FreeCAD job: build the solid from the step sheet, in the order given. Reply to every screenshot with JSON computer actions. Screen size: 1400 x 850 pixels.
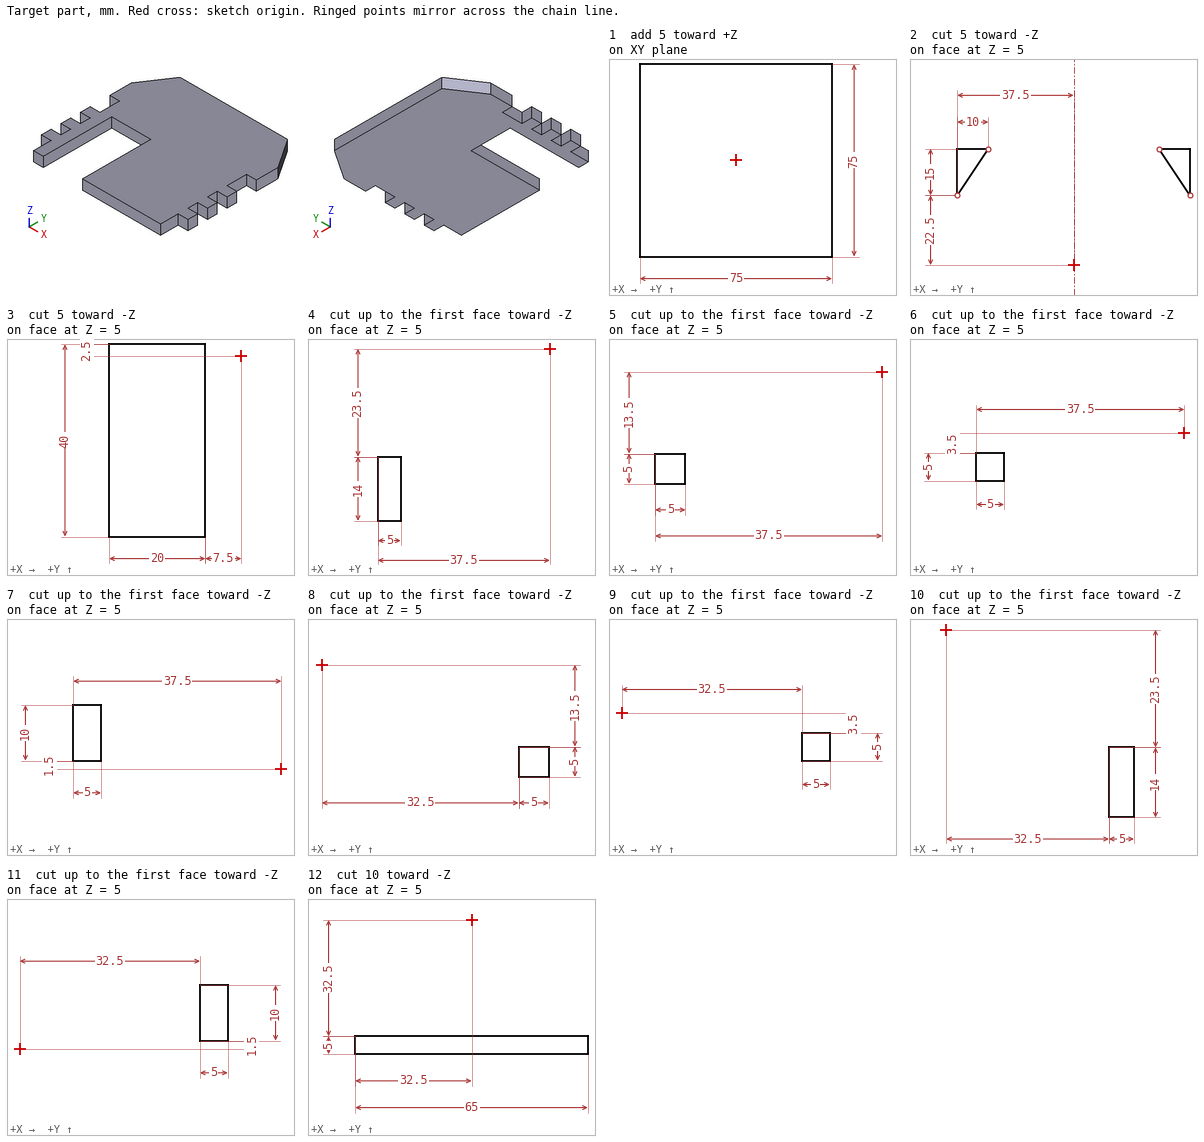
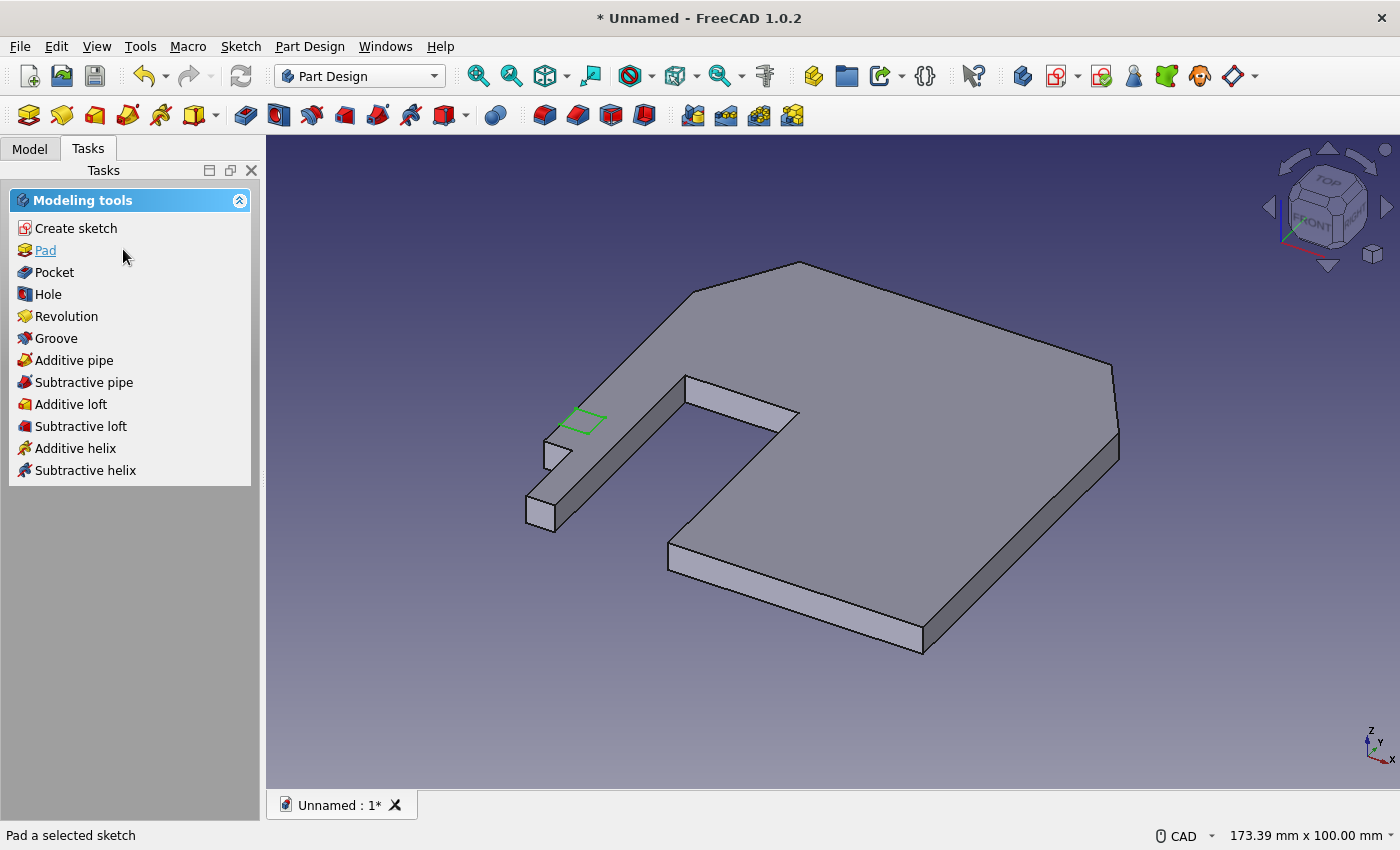
{"action": "left_click", "coordinate": [246, 116]}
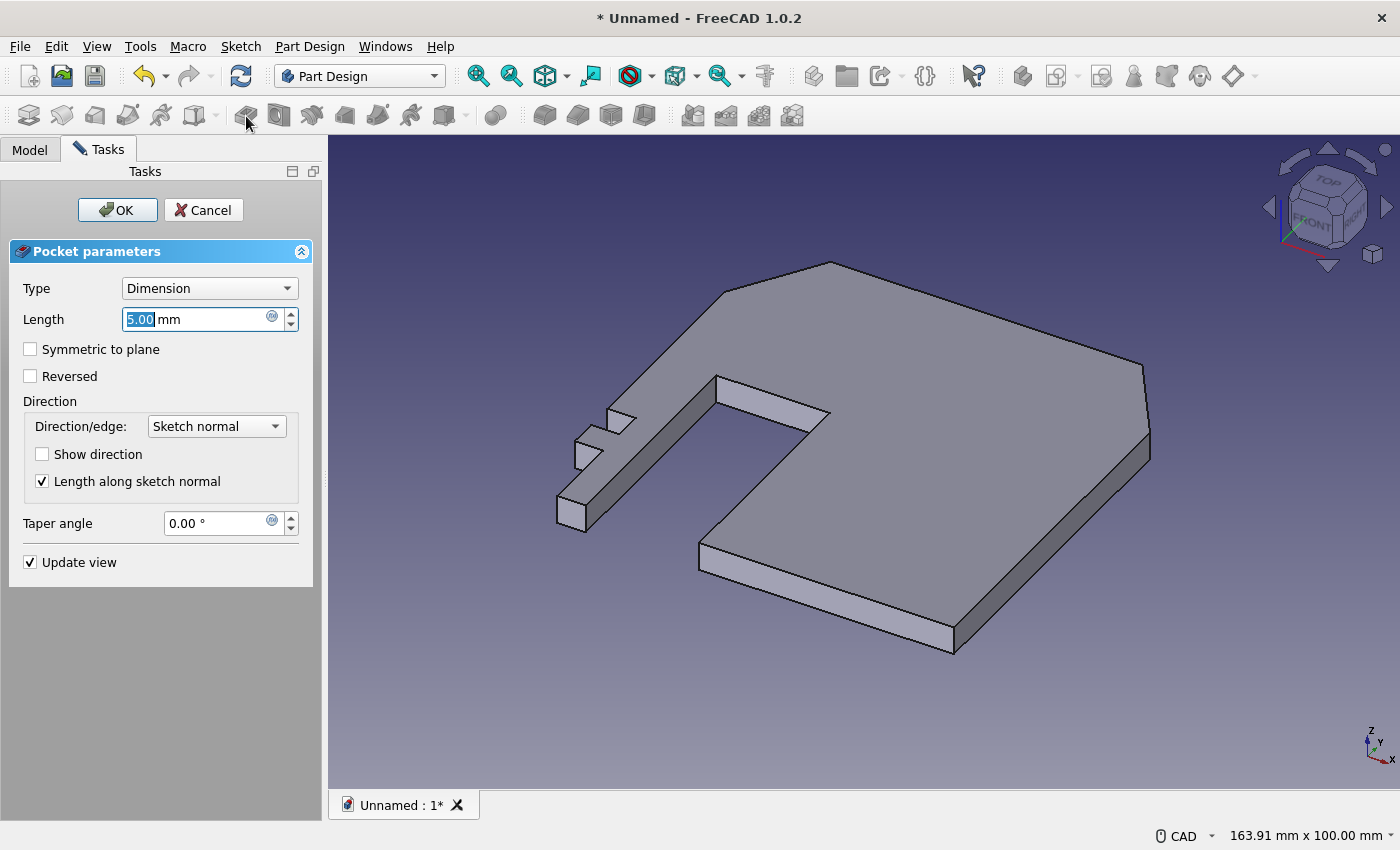
{"action": "left_click", "coordinate": [210, 288]}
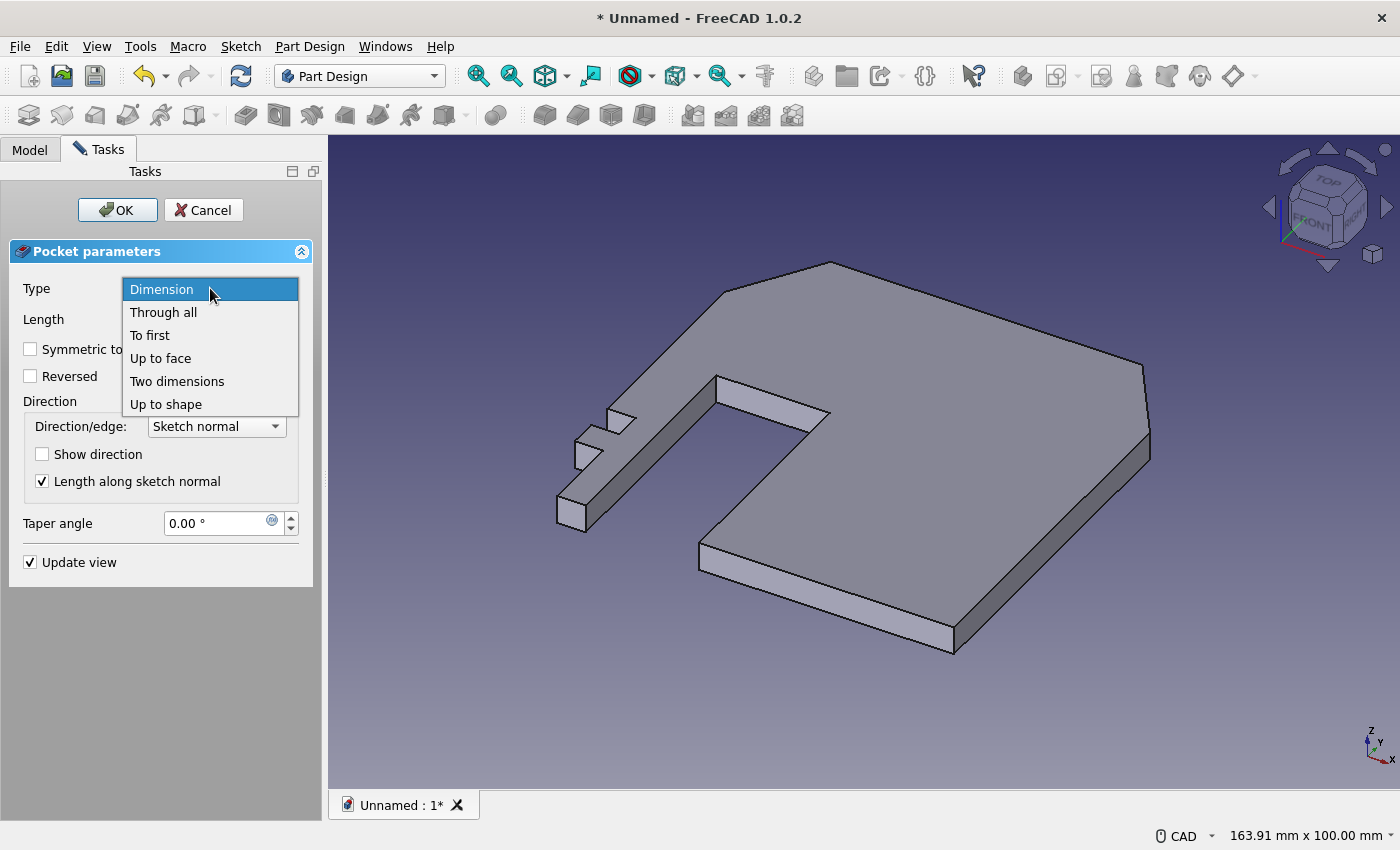
{"action": "left_click", "coordinate": [208, 336]}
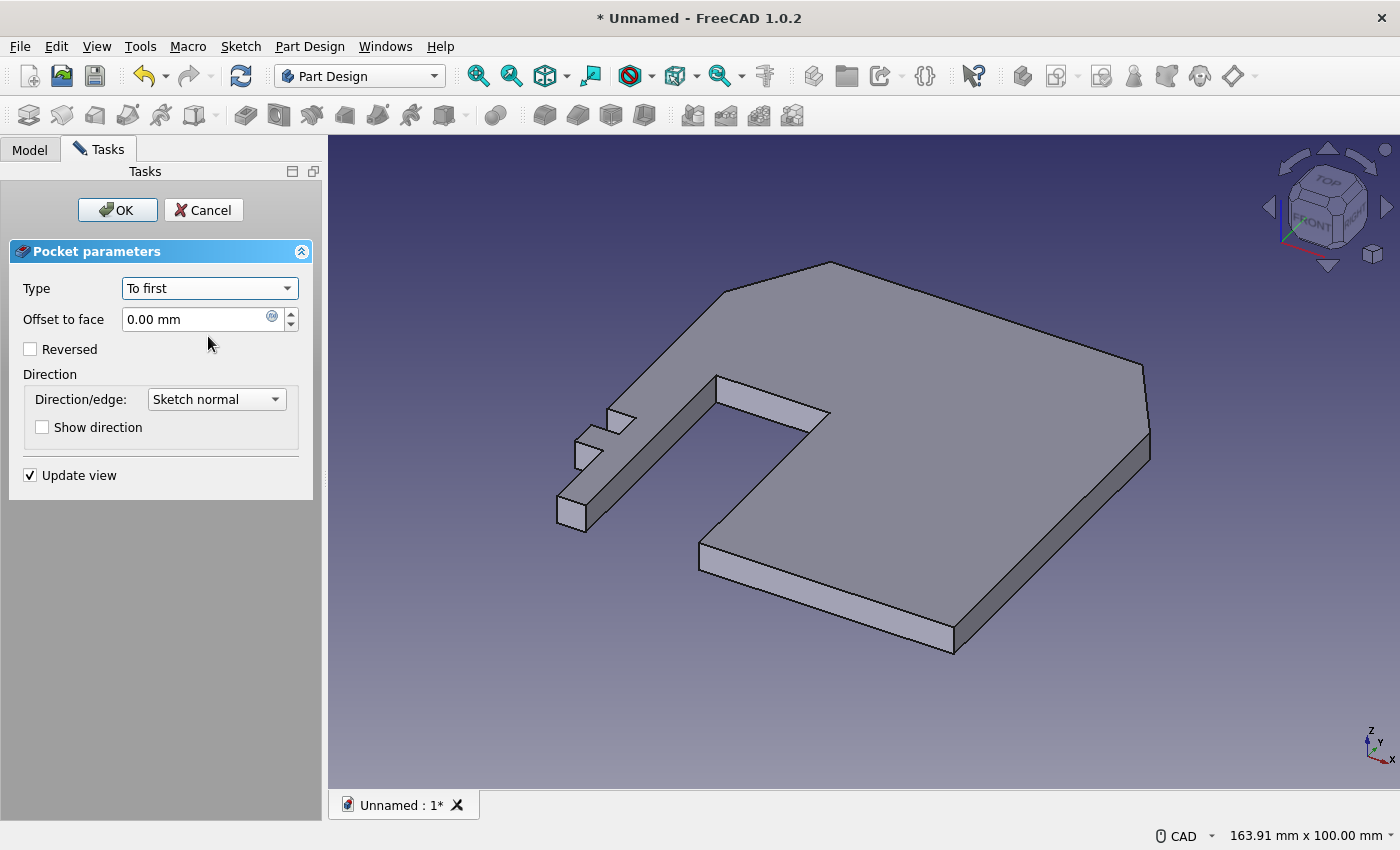
{"action": "left_click", "coordinate": [118, 210]}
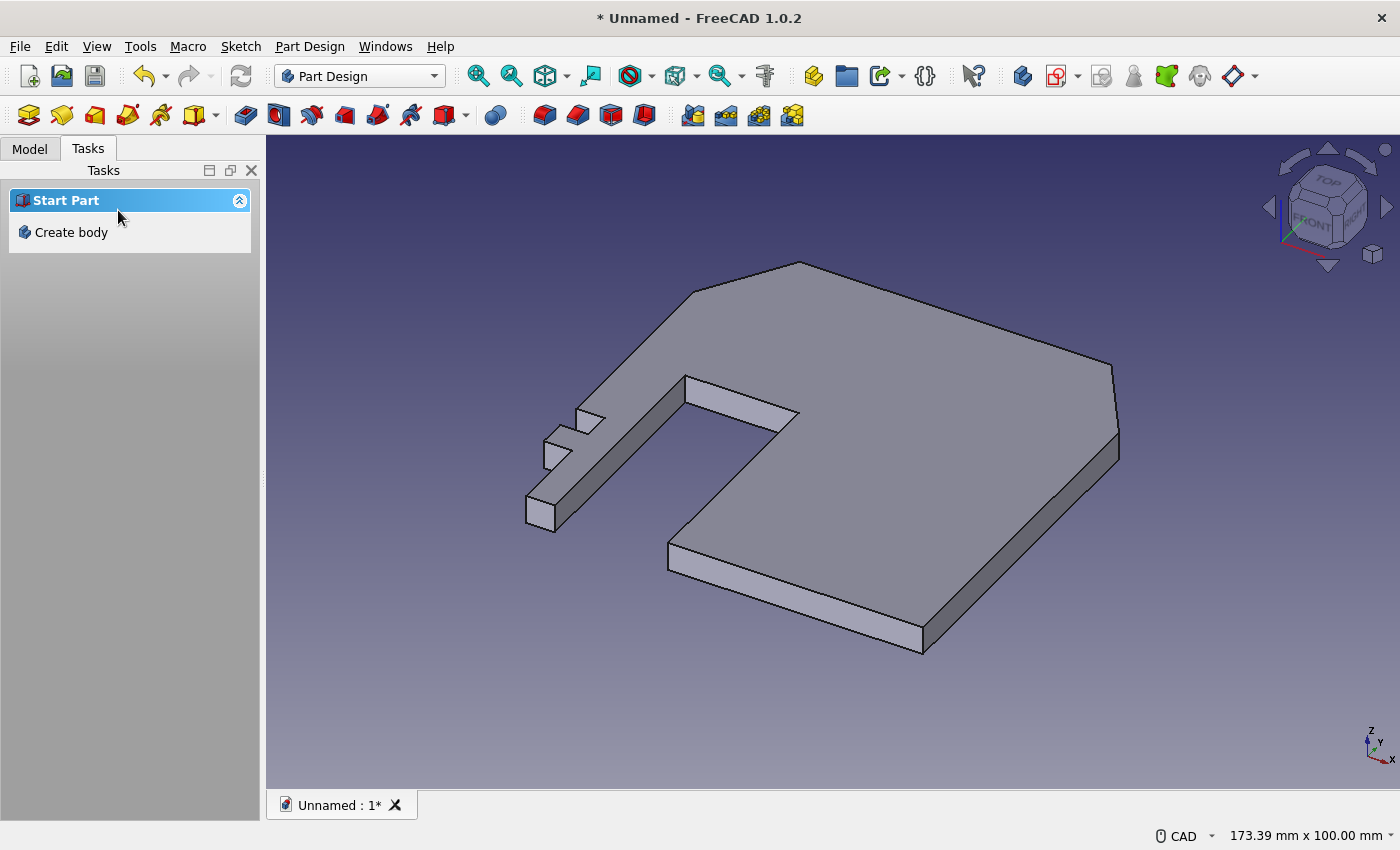
{"action": "left_click", "coordinate": [929, 420]}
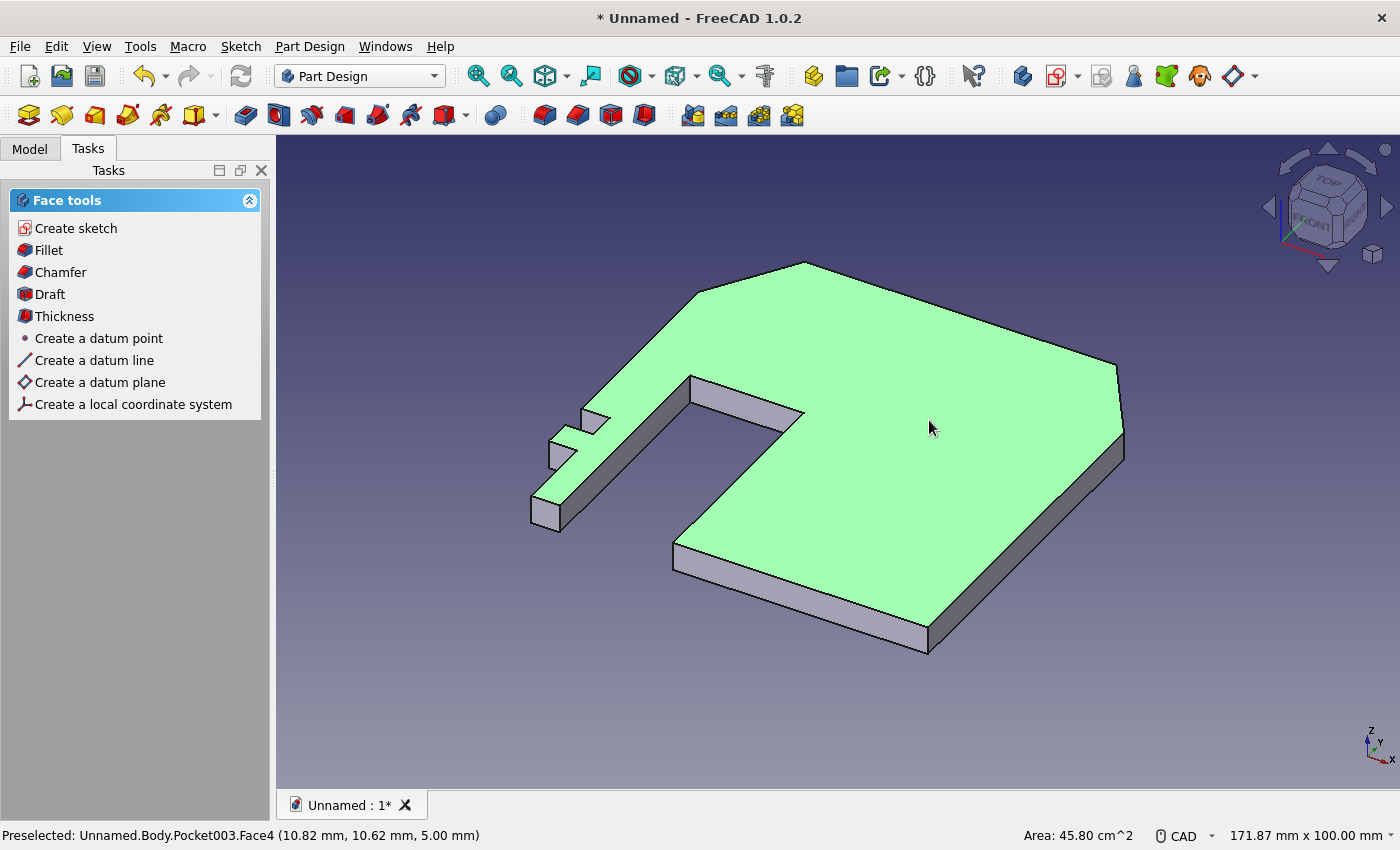
{"action": "left_click", "coordinate": [1056, 76]}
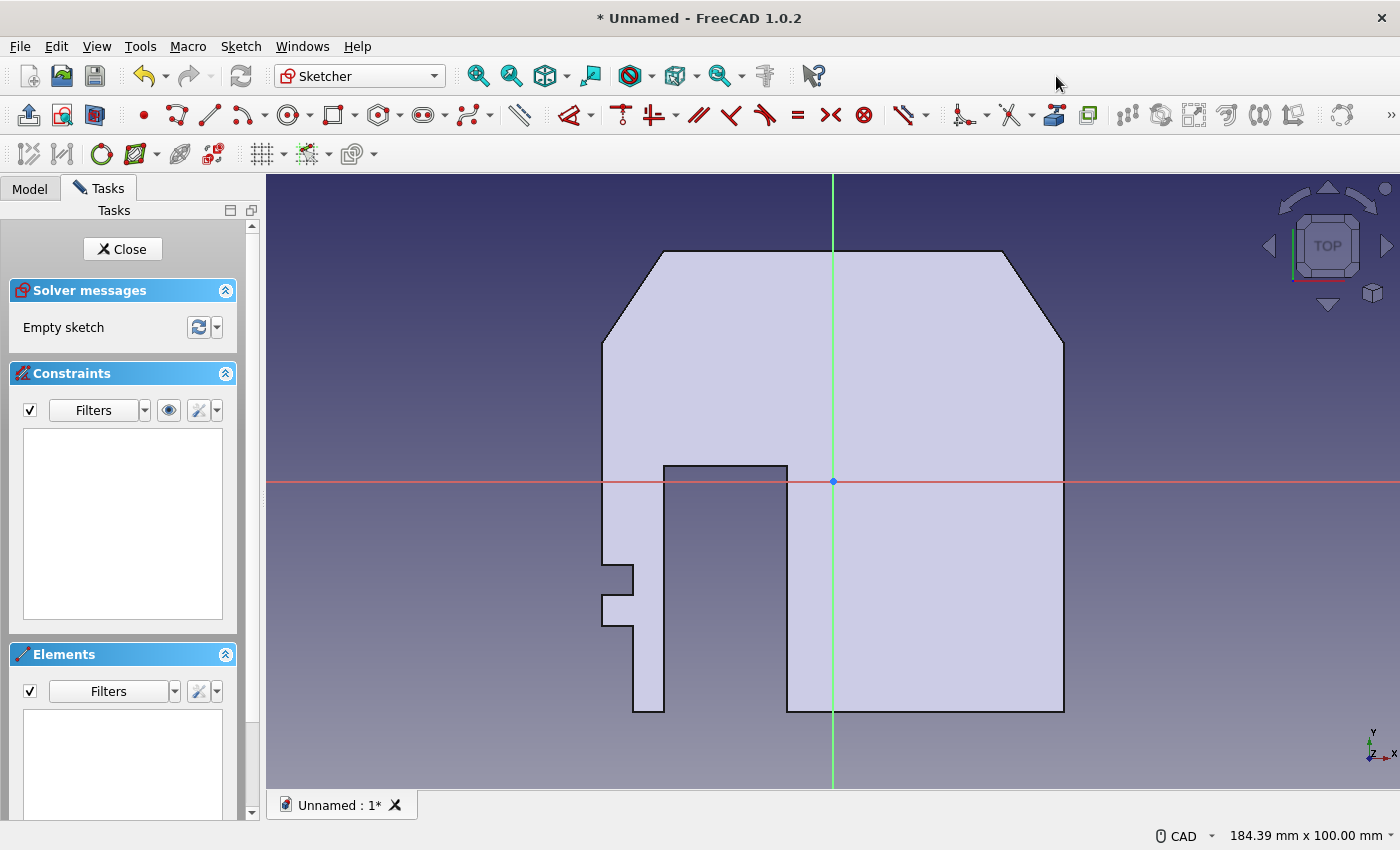
{"action": "scroll", "coordinate": [606, 521], "scroll_direction": "up", "scroll_amount": 13}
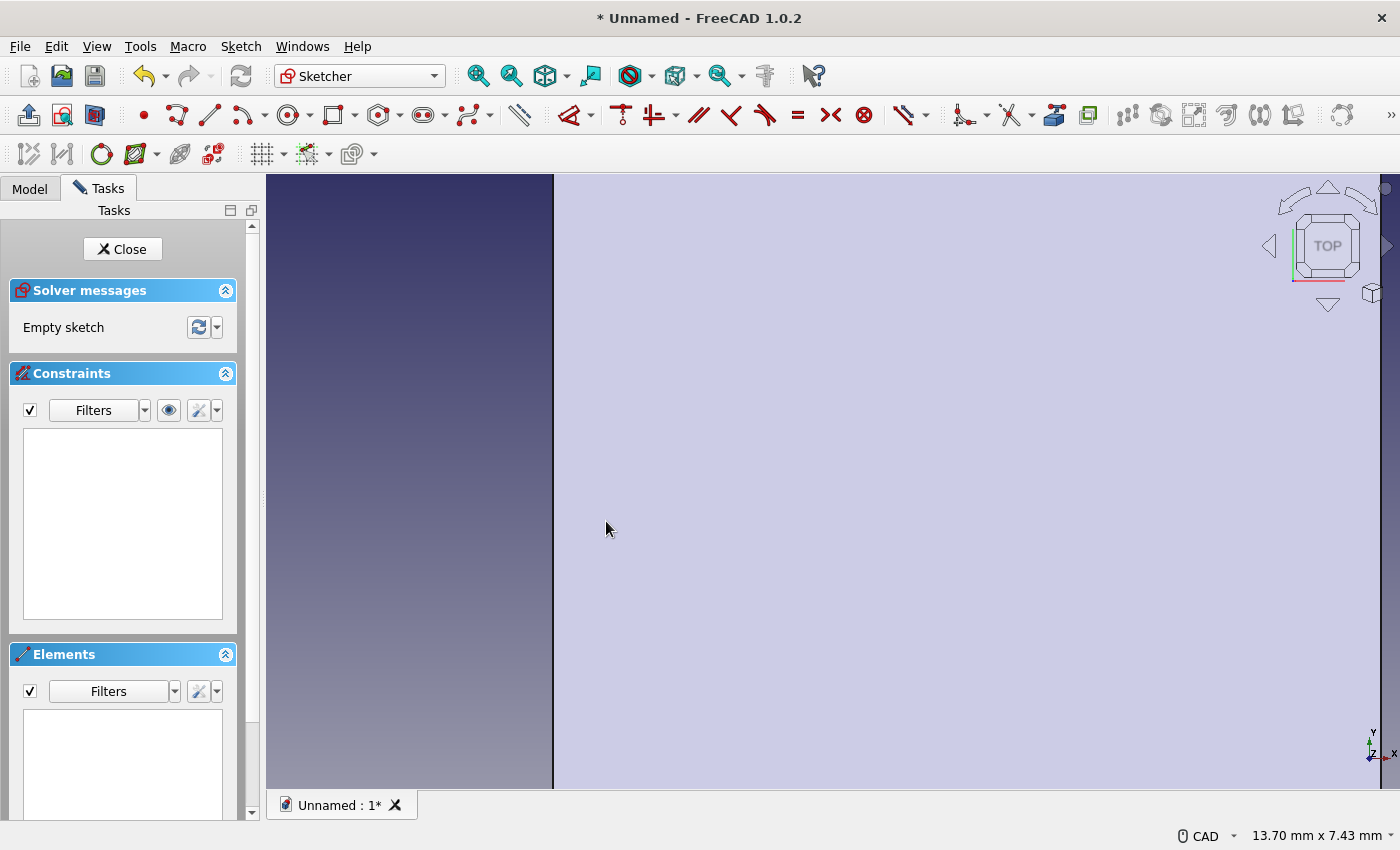
{"action": "key", "text": "g r"}